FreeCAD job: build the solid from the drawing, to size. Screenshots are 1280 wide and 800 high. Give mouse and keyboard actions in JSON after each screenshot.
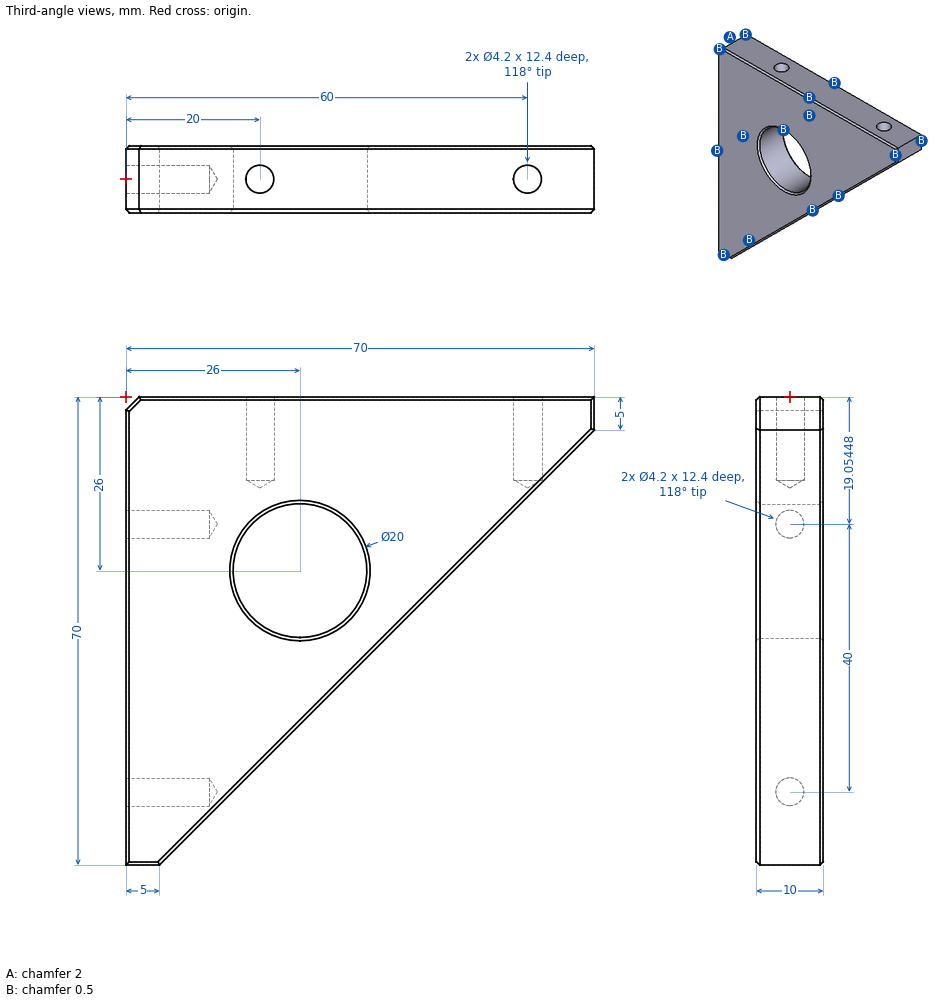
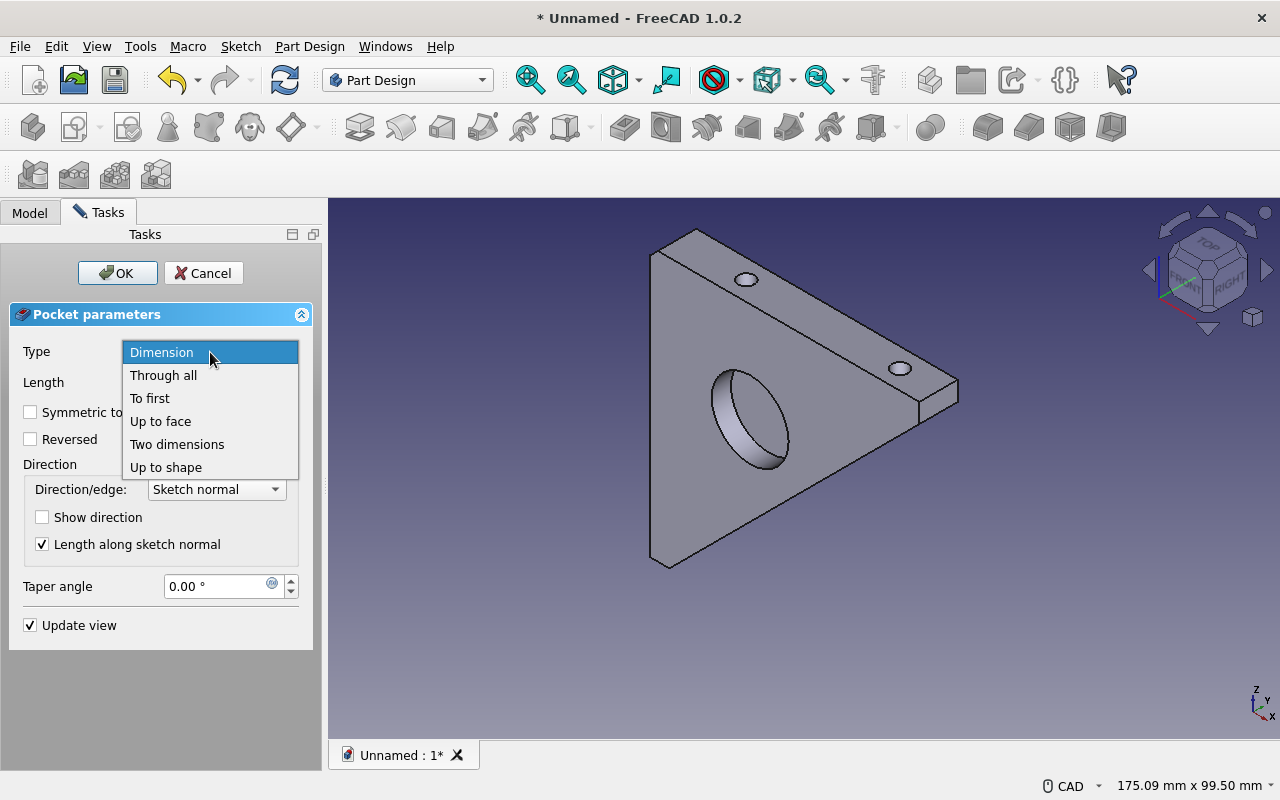
{"action": "left_click", "coordinate": [208, 376]}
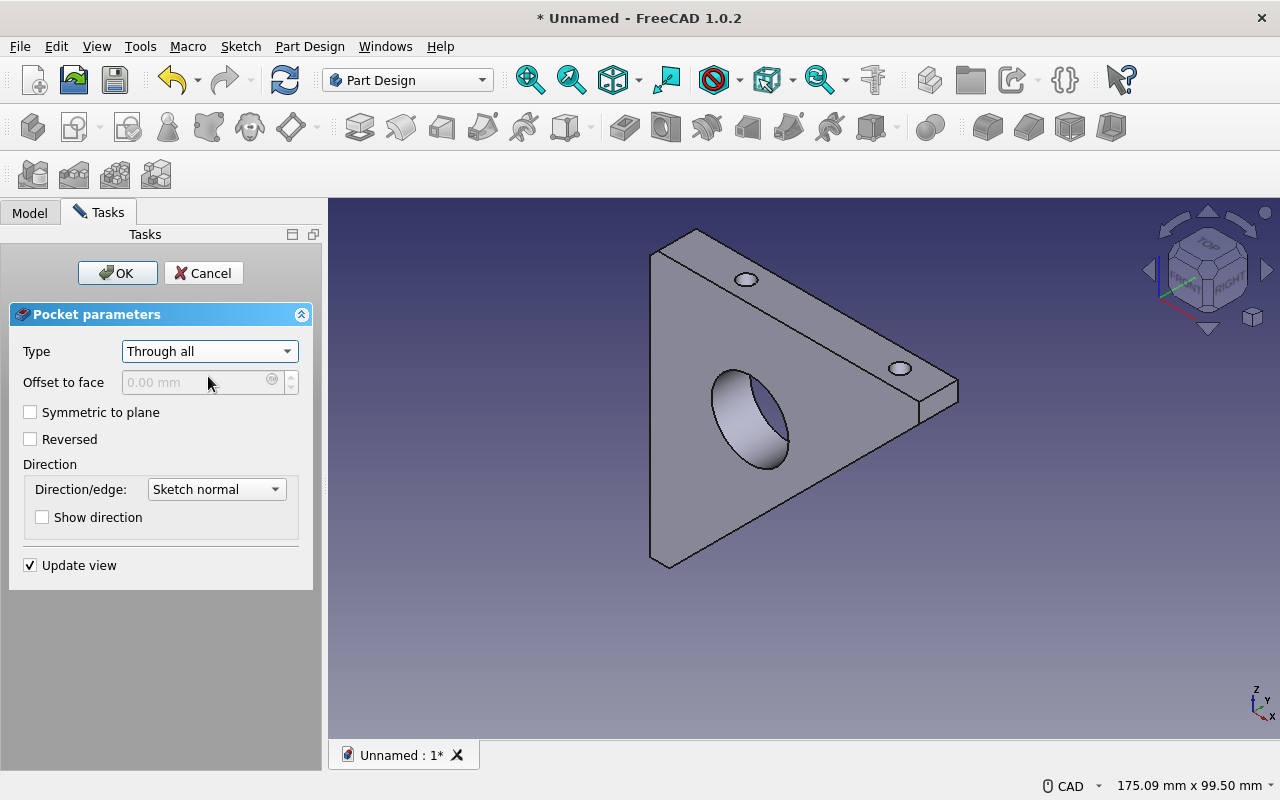
{"action": "left_click", "coordinate": [118, 273]}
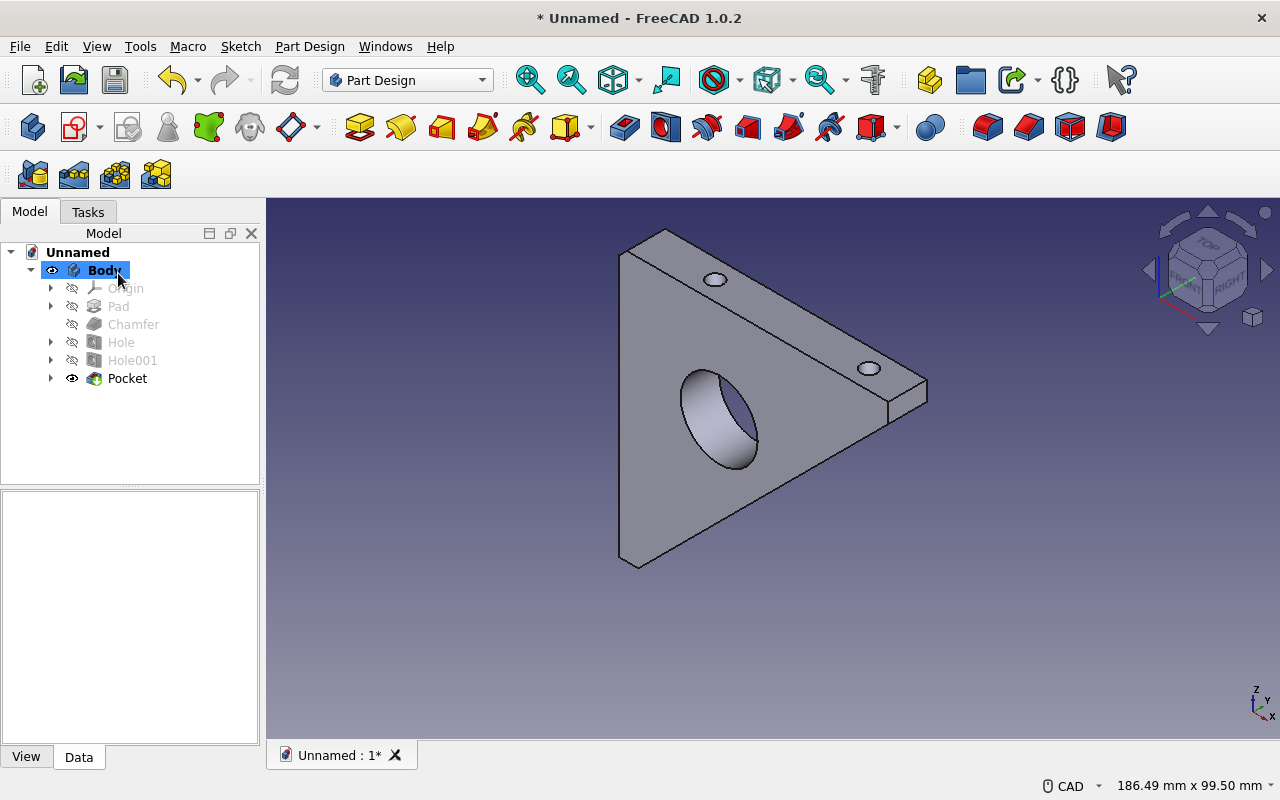
{"action": "left_click", "coordinate": [792, 412]}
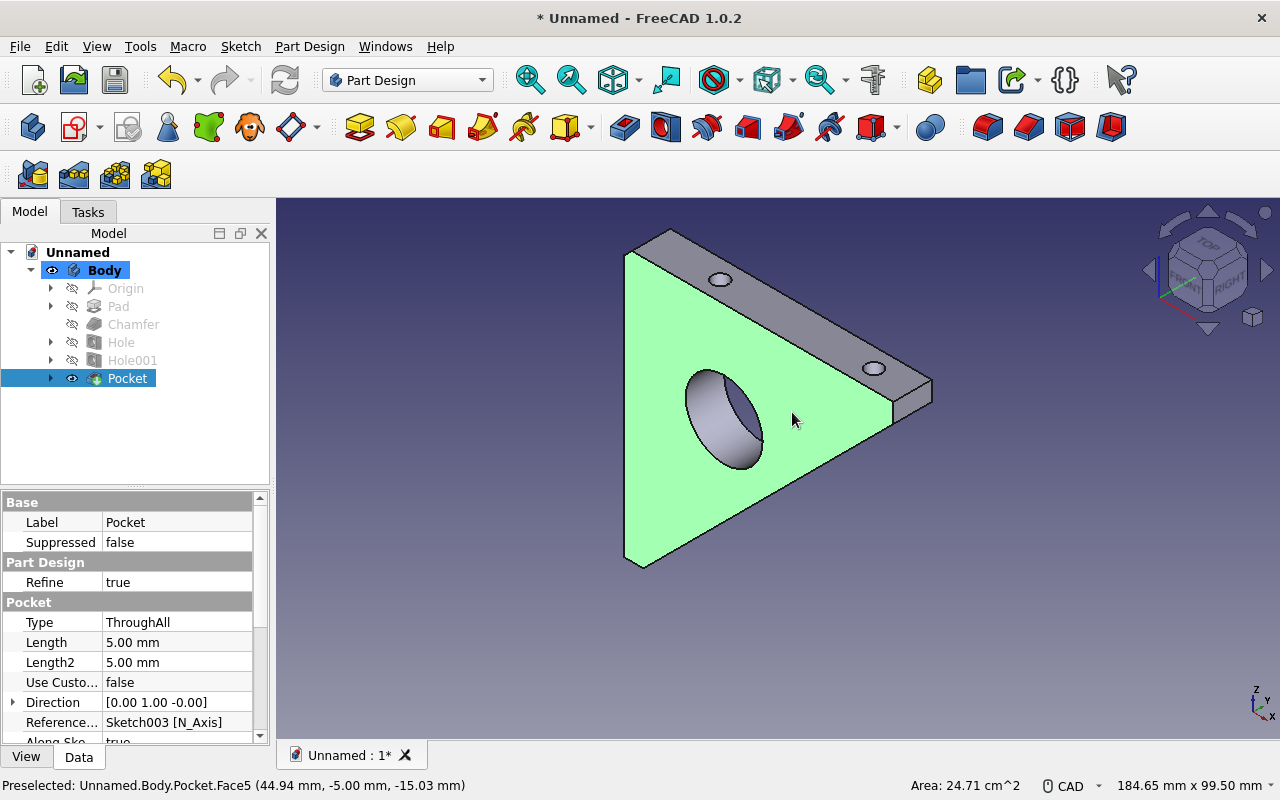
{"action": "key", "text": "2"}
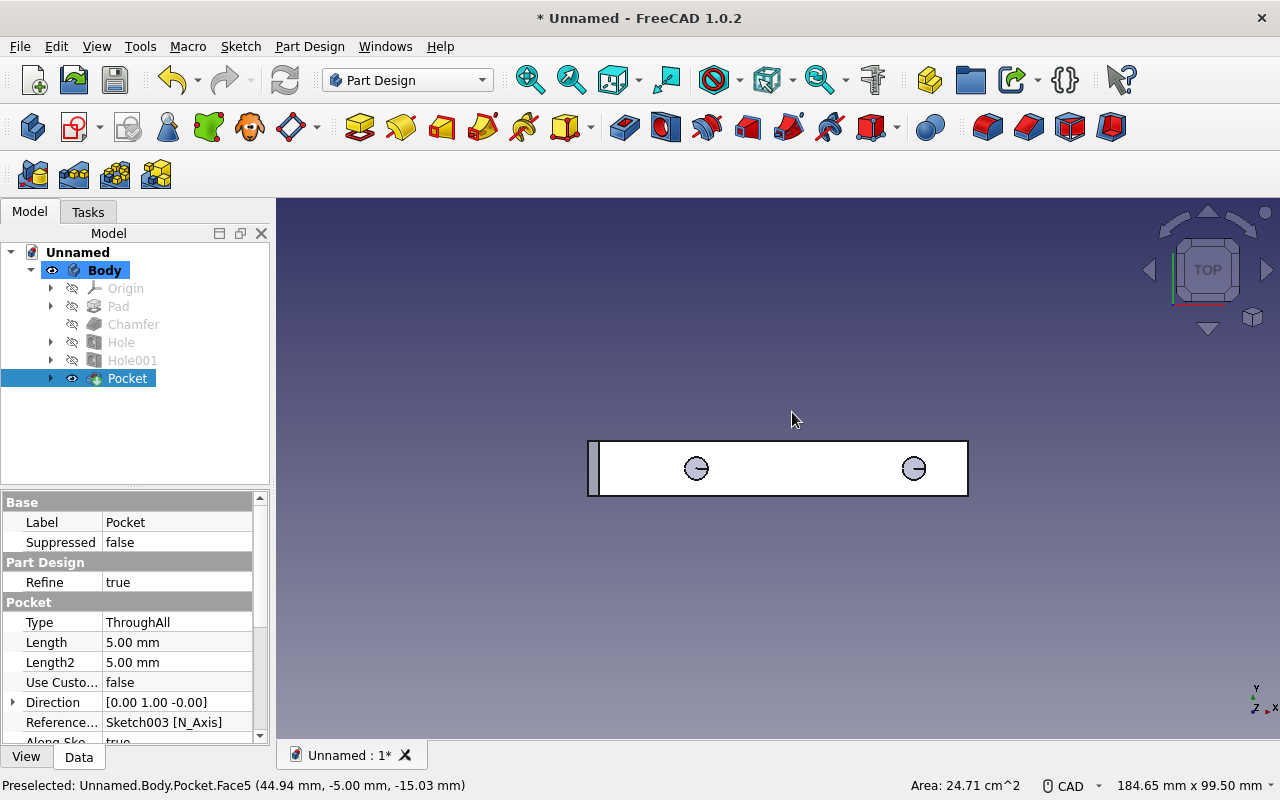
{"action": "left_click", "coordinate": [531, 80]}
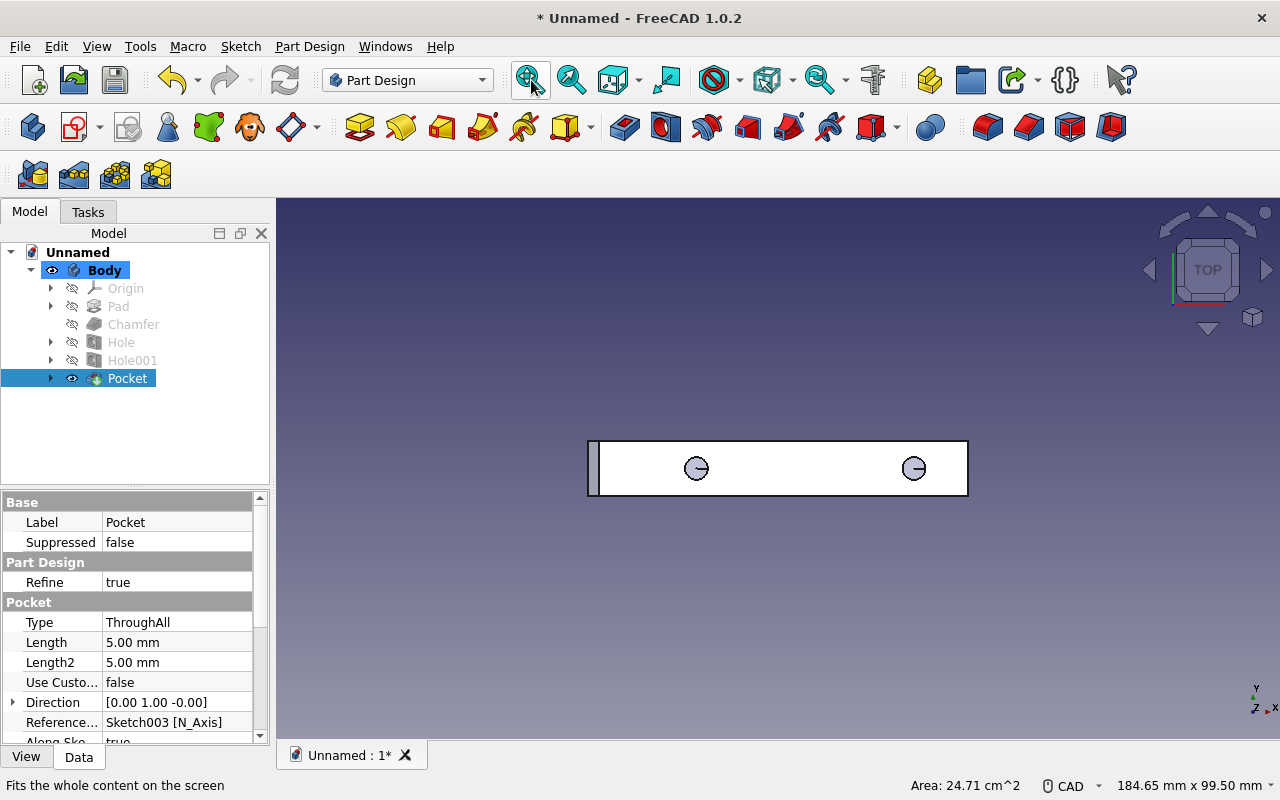
{"action": "key", "text": "0"}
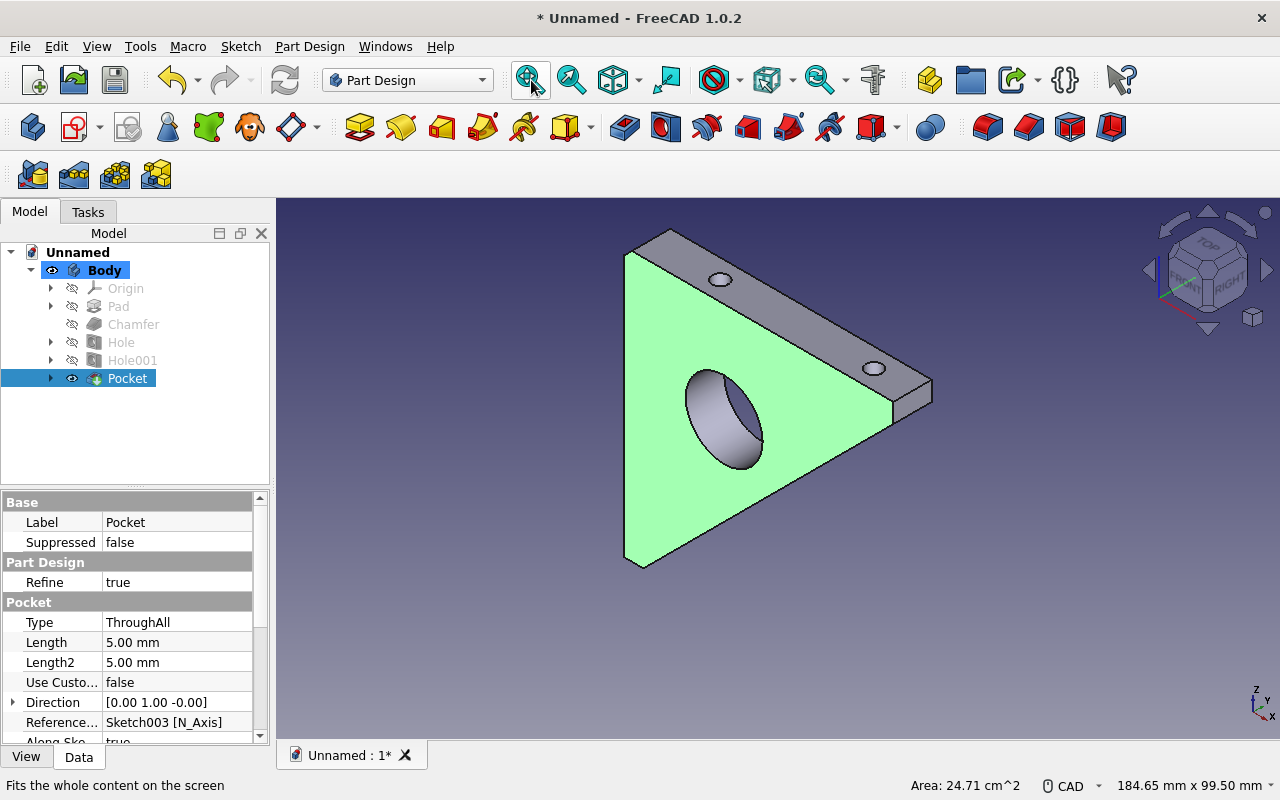
{"action": "key", "text": "1"}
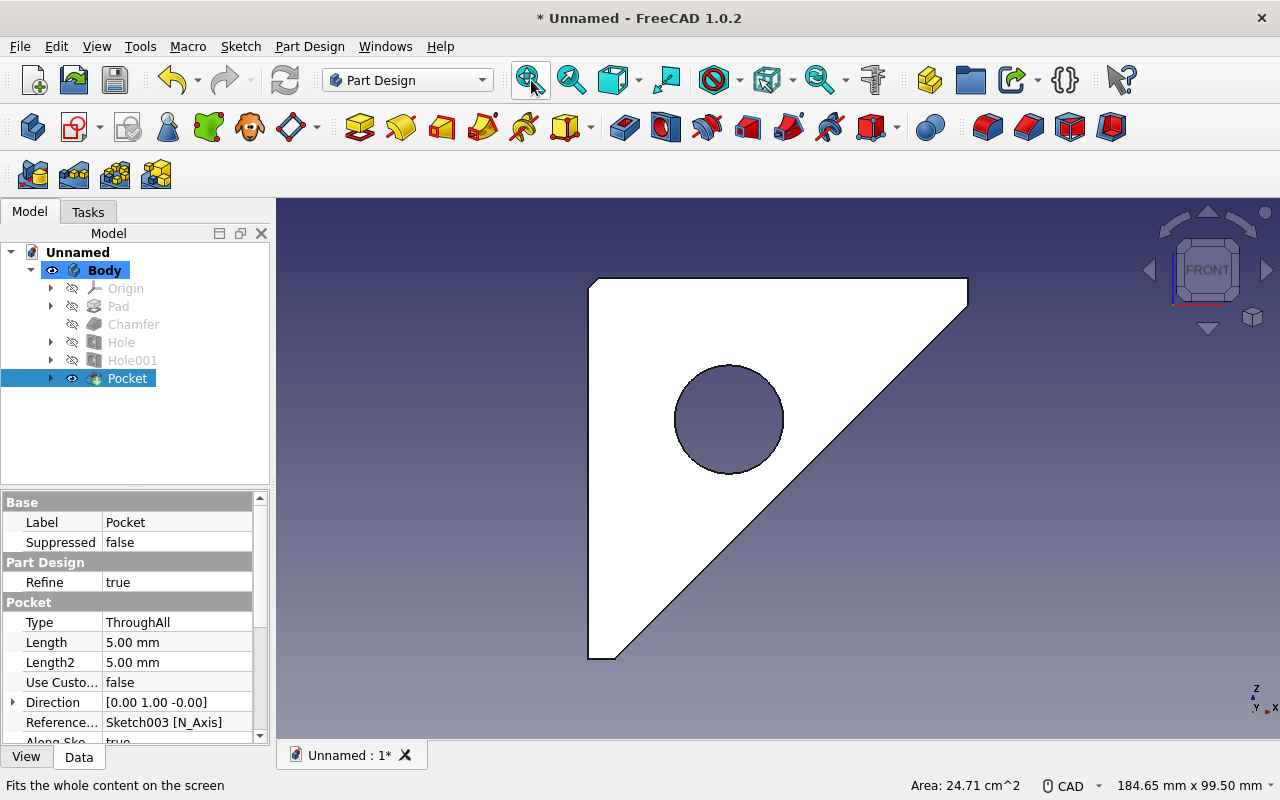
{"action": "key", "text": "3"}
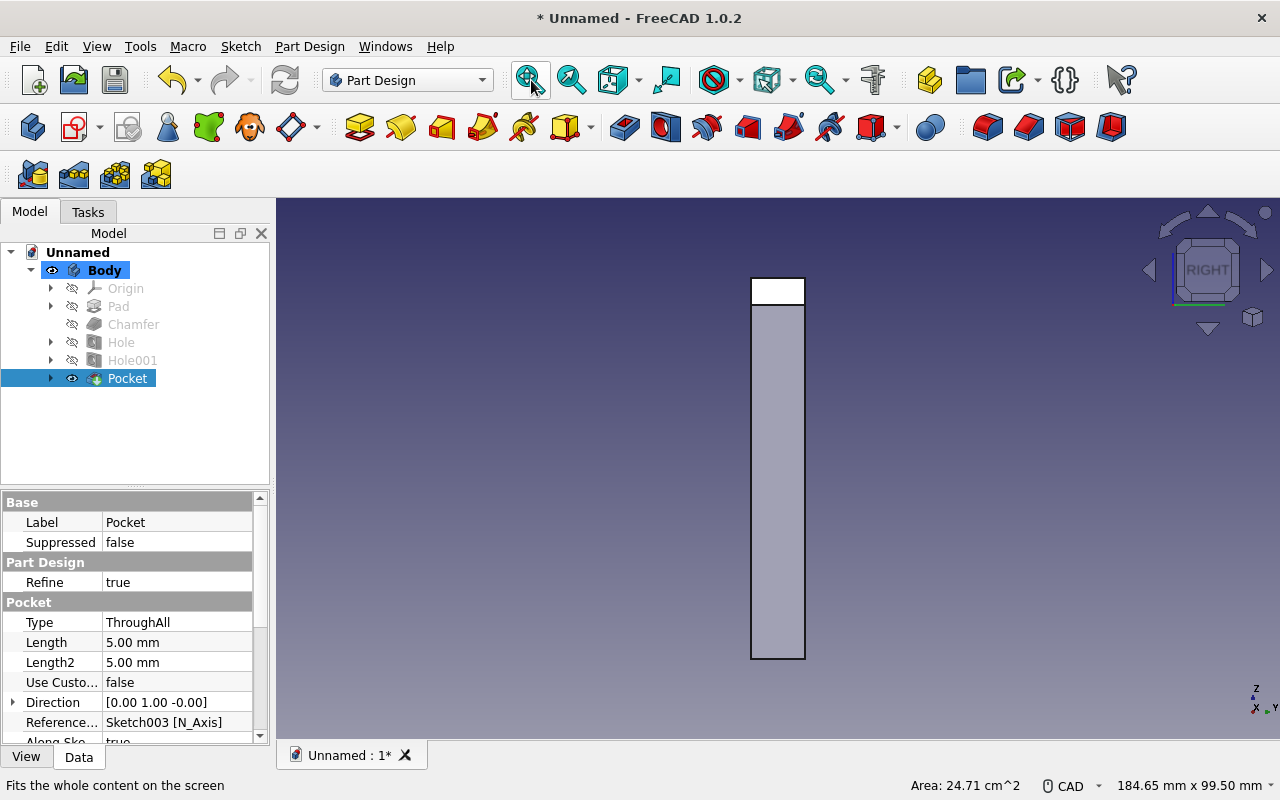
{"action": "key", "text": "5"}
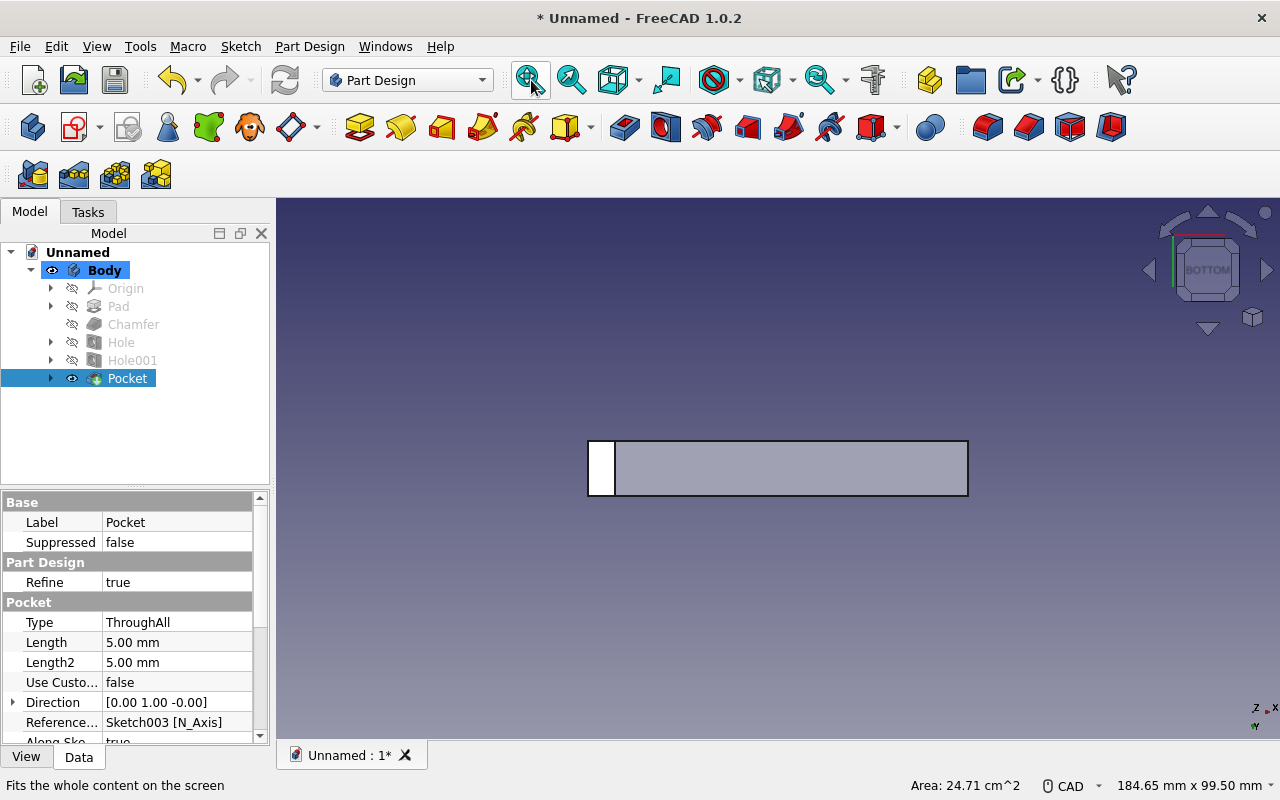
{"action": "left_click", "coordinate": [531, 80]}